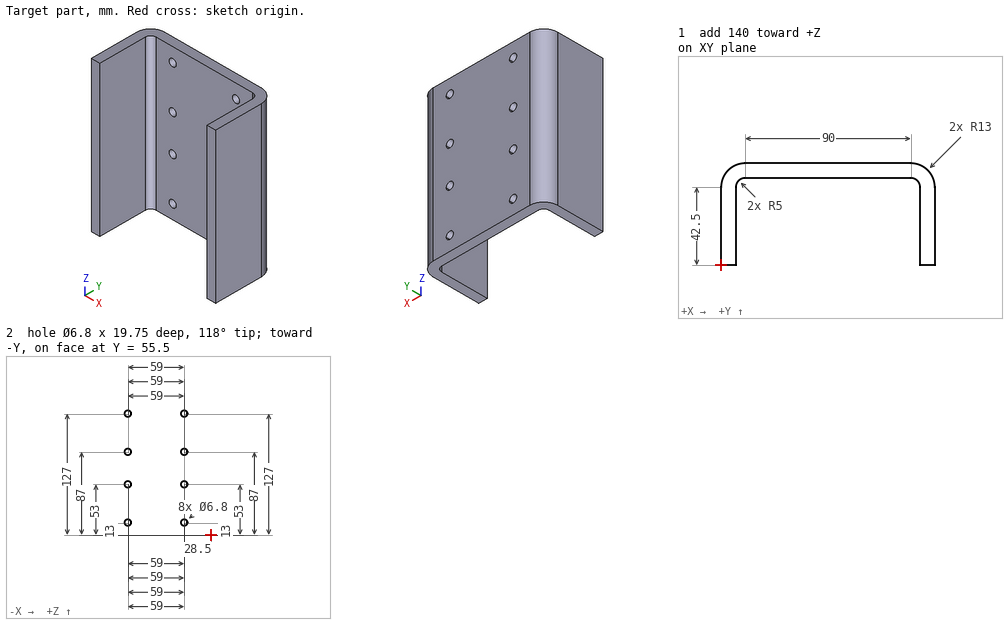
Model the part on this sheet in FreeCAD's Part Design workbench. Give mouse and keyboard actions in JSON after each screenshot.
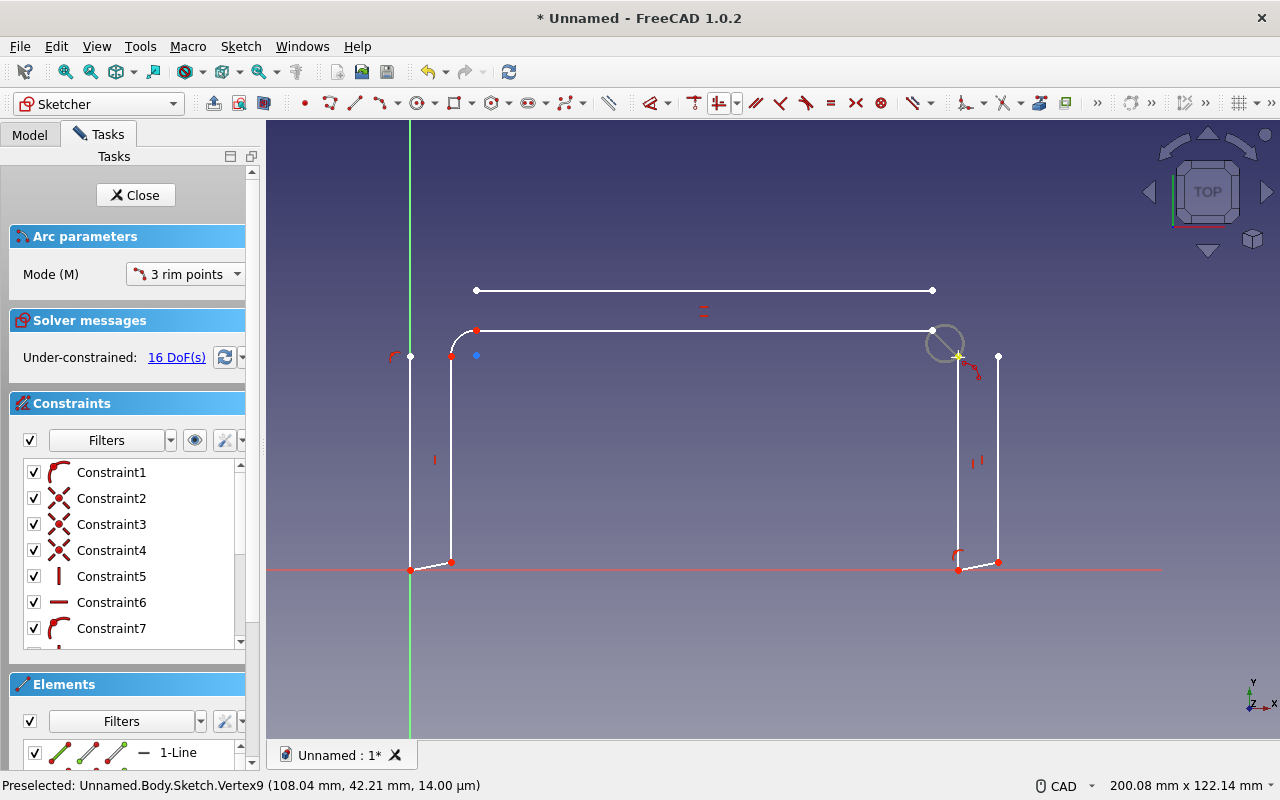
{"action": "scroll", "coordinate": [950, 337], "scroll_direction": "up", "scroll_amount": 4}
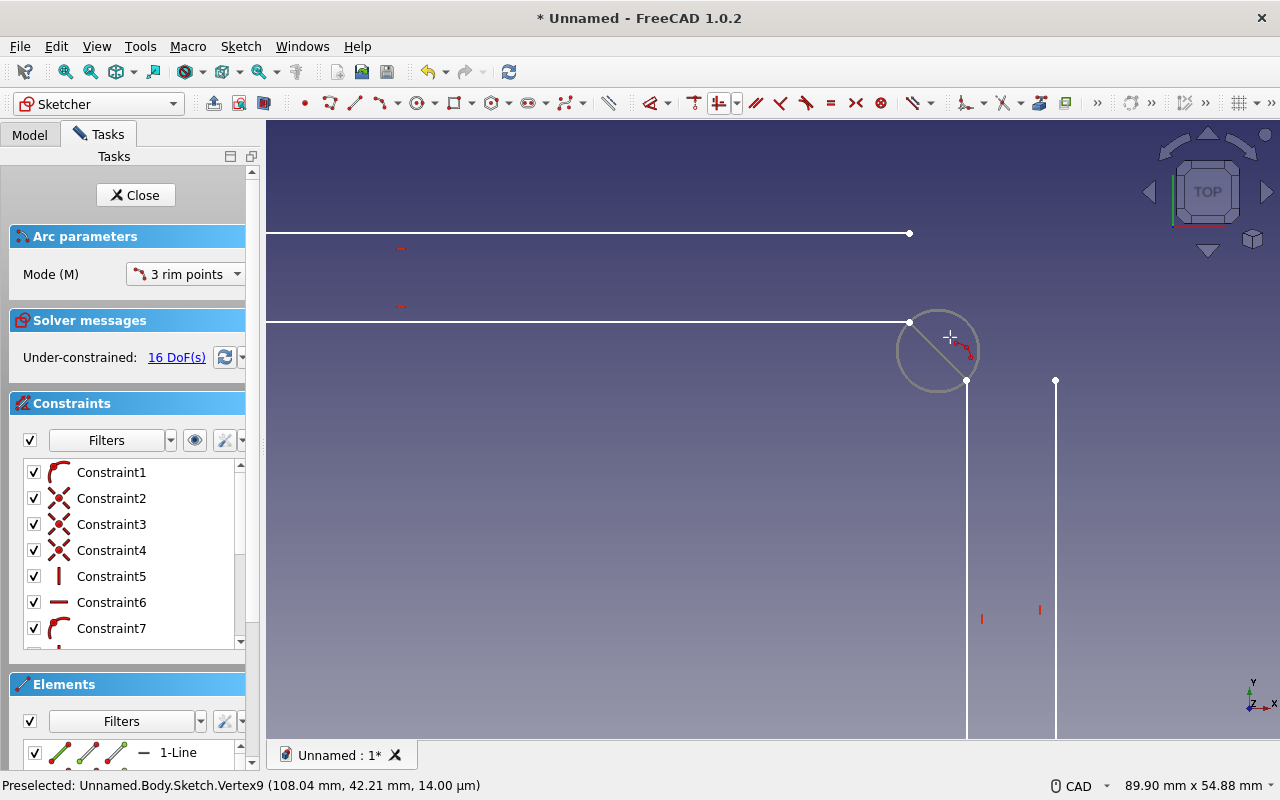
{"action": "left_click", "coordinate": [950, 337]}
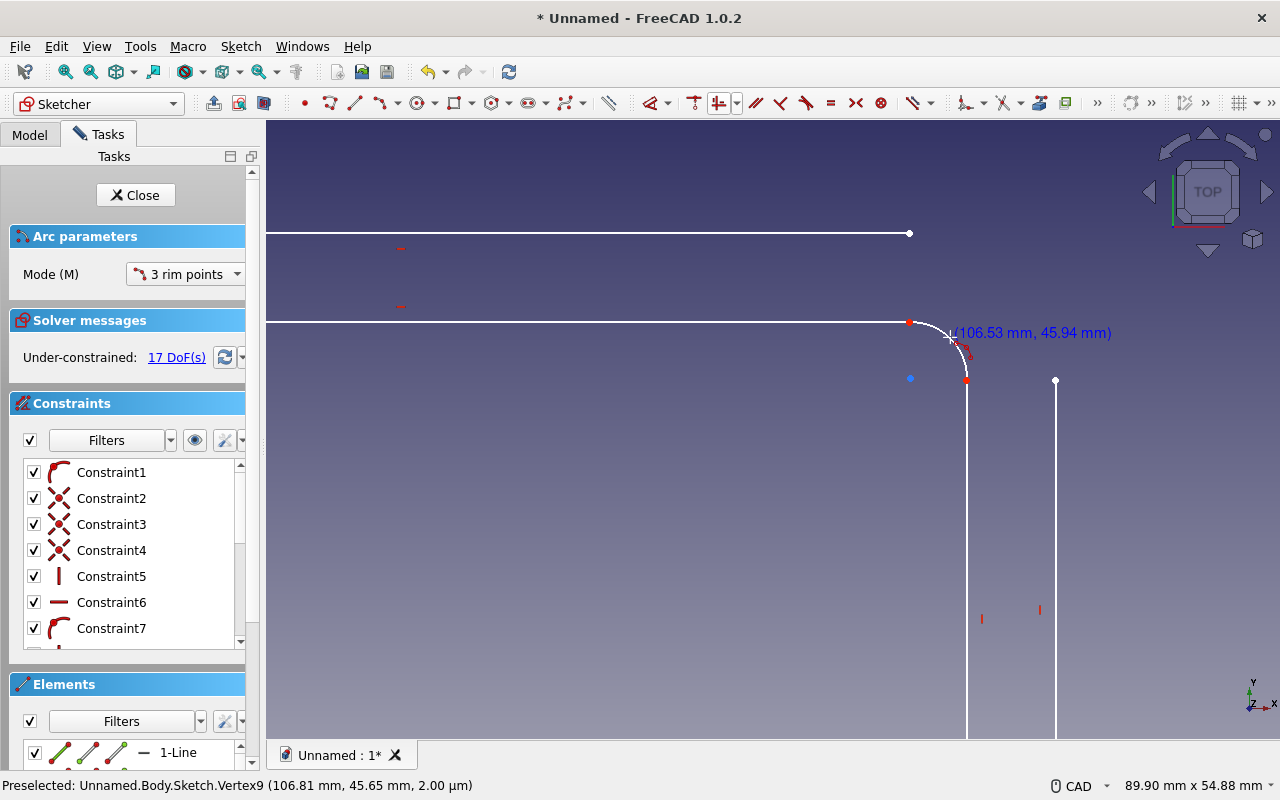
{"action": "left_click", "coordinate": [1056, 380]}
{"action": "left_click", "coordinate": [909, 233]}
{"action": "left_click", "coordinate": [1014, 273]}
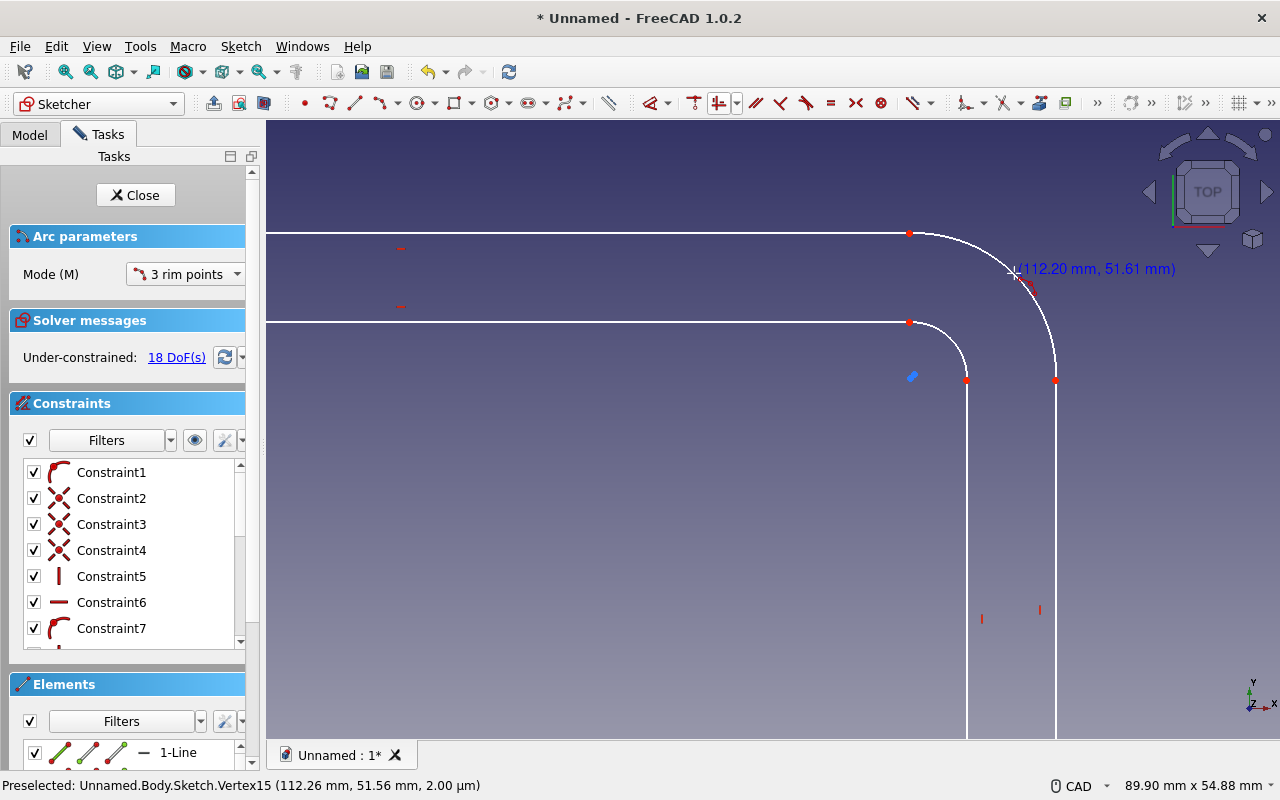
{"action": "scroll", "coordinate": [951, 337], "scroll_direction": "down", "scroll_amount": 4}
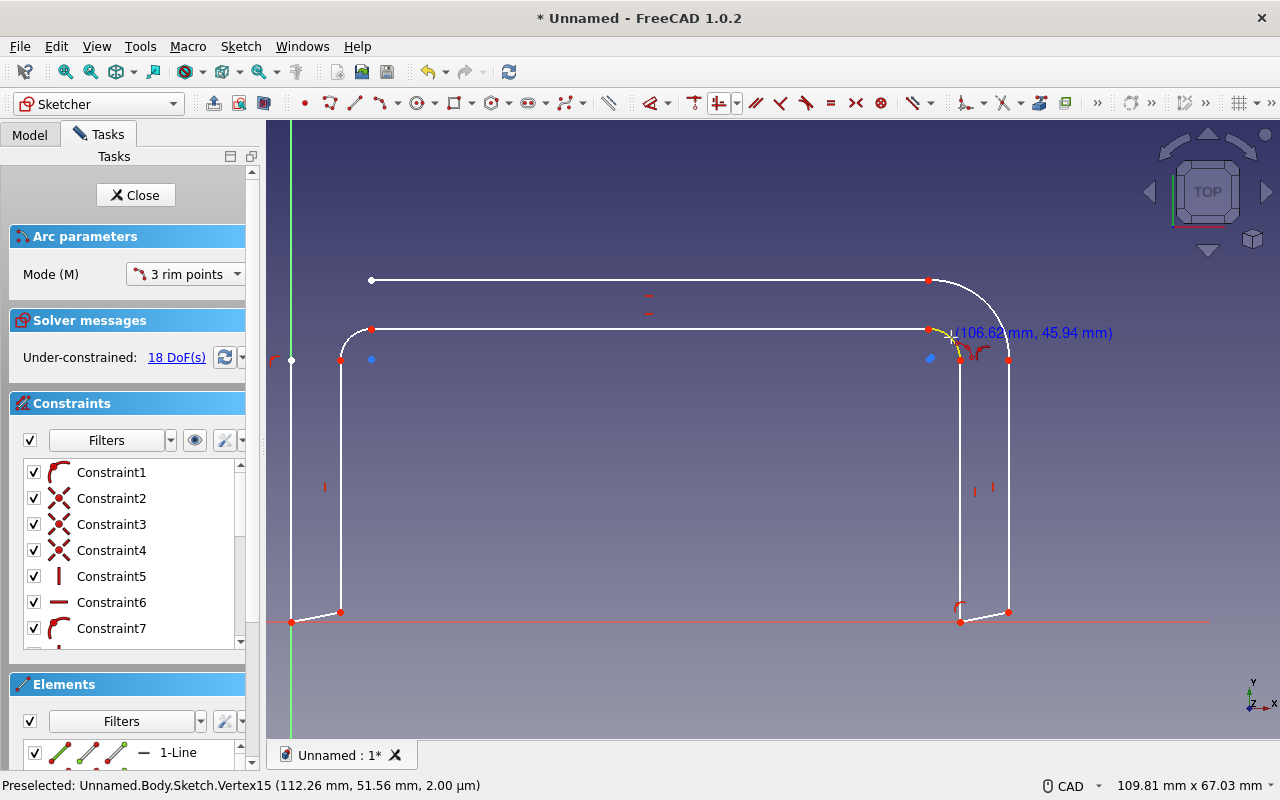
{"action": "left_click", "coordinate": [477, 291]}
{"action": "left_click", "coordinate": [411, 357]}
{"action": "left_click", "coordinate": [430, 308]}
{"action": "key", "text": "Escape"}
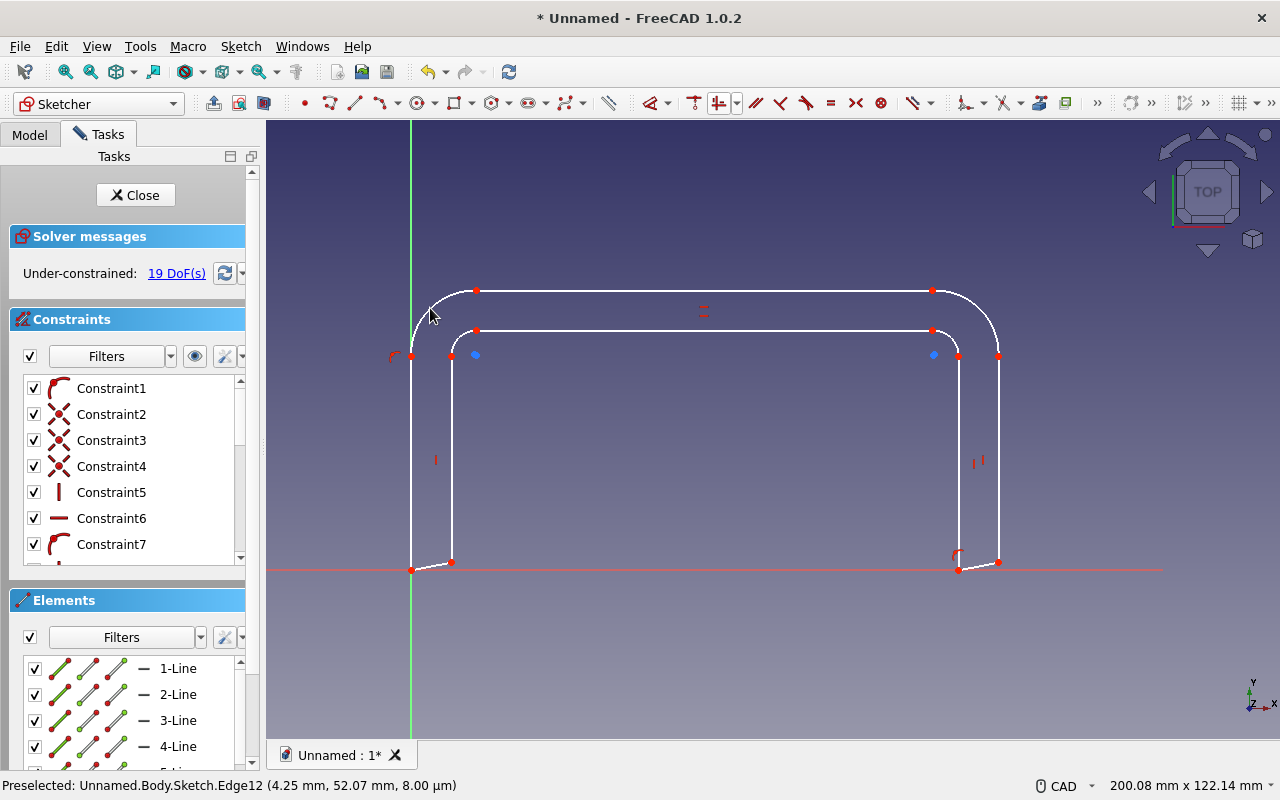
{"action": "left_click", "coordinate": [411, 421]}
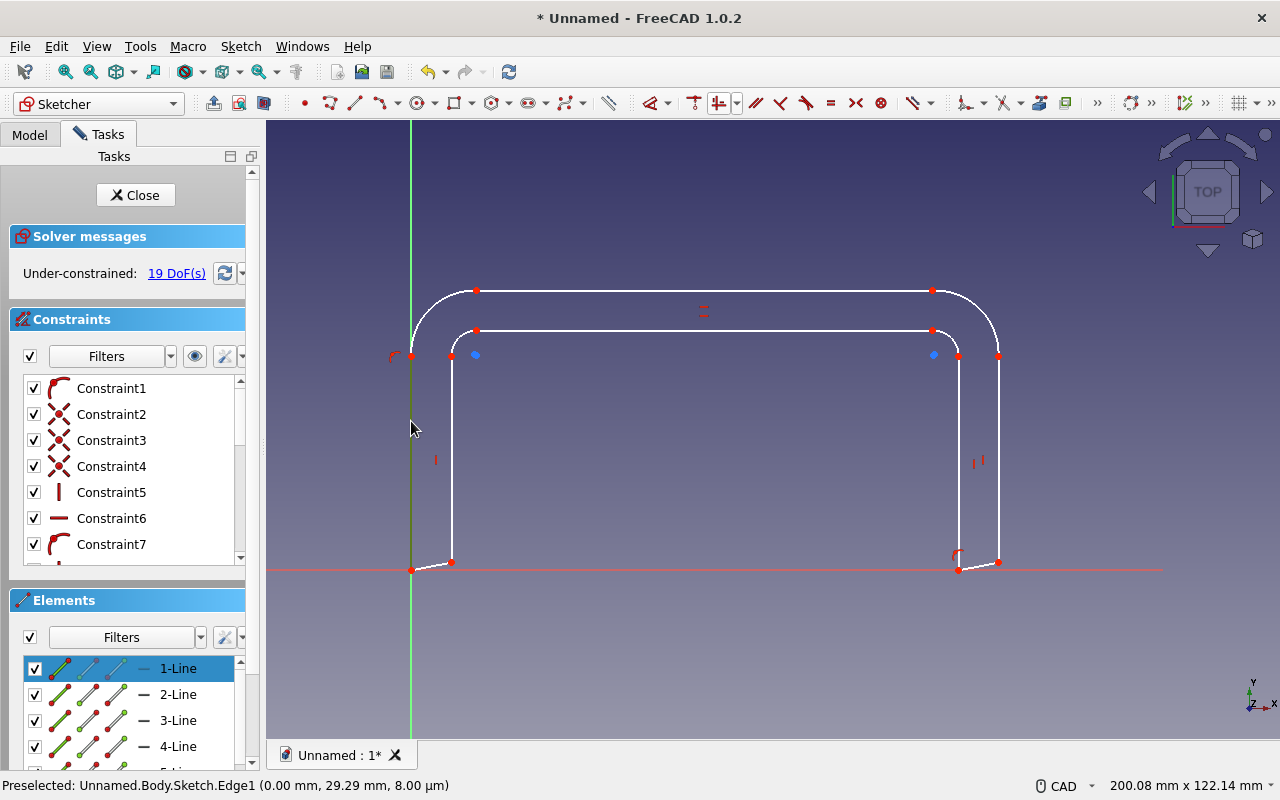
{"action": "left_click", "coordinate": [446, 297]}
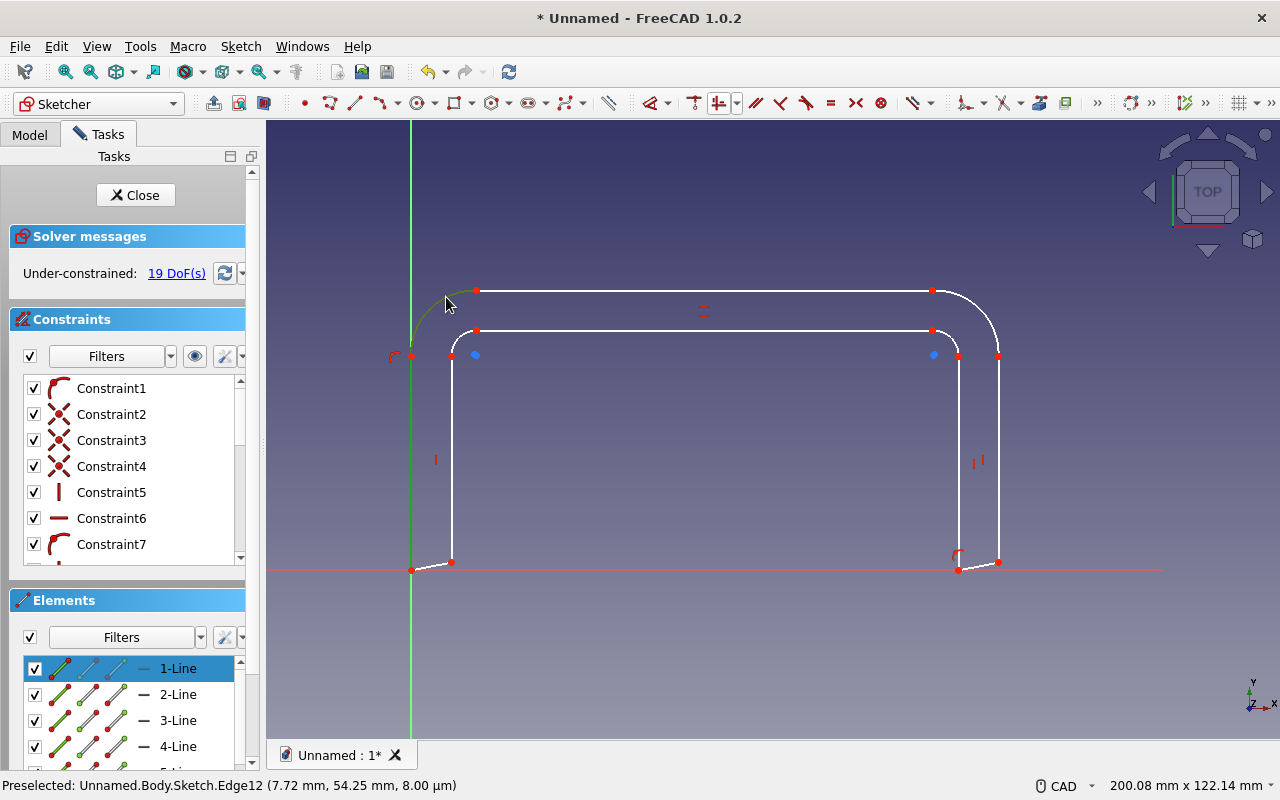
{"action": "key", "text": "t"}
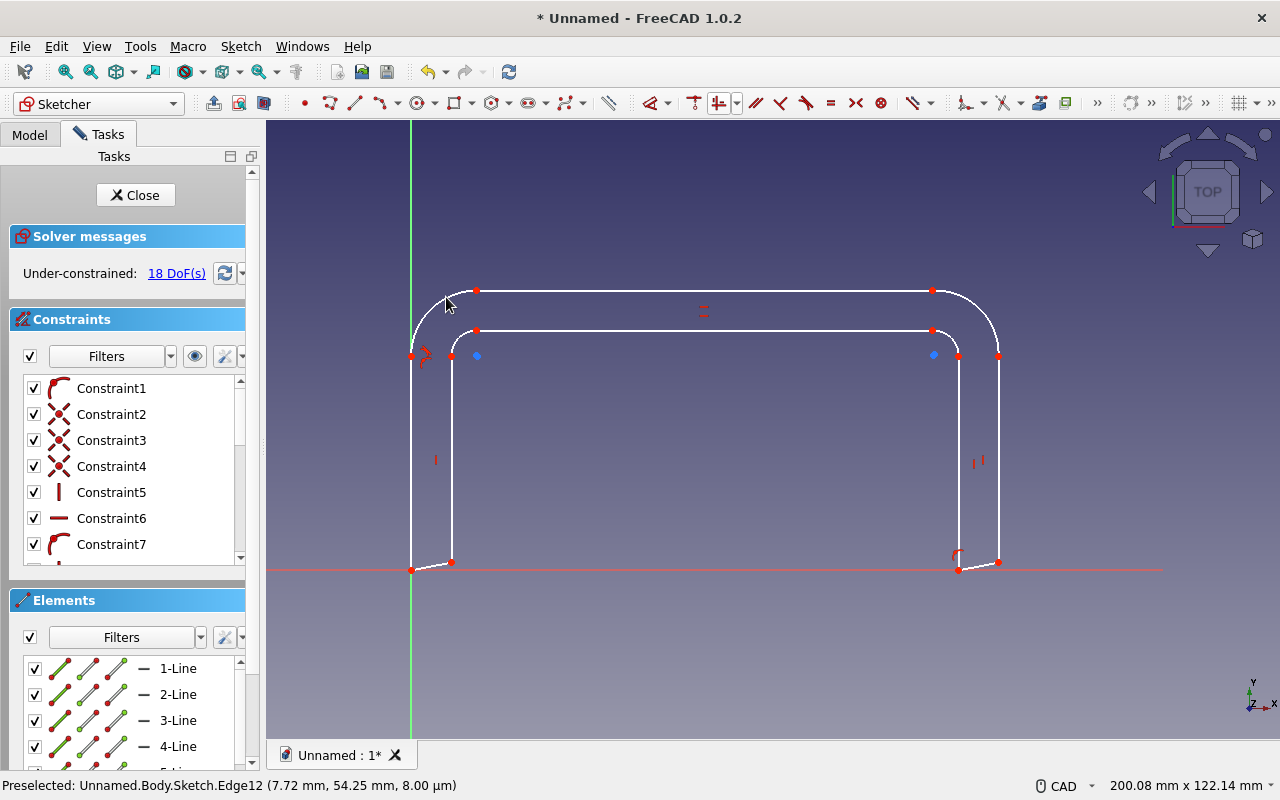
{"action": "left_click", "coordinate": [452, 501]}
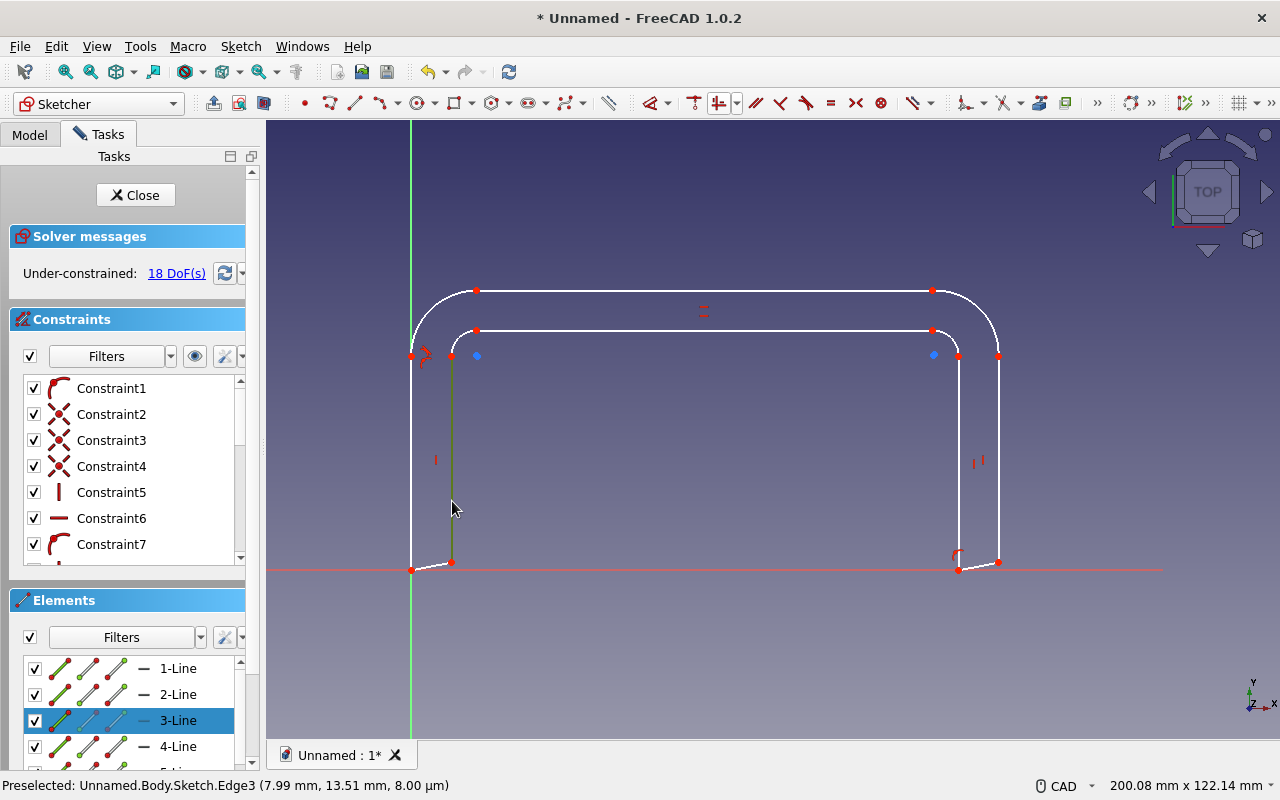
{"action": "left_click", "coordinate": [465, 333]}